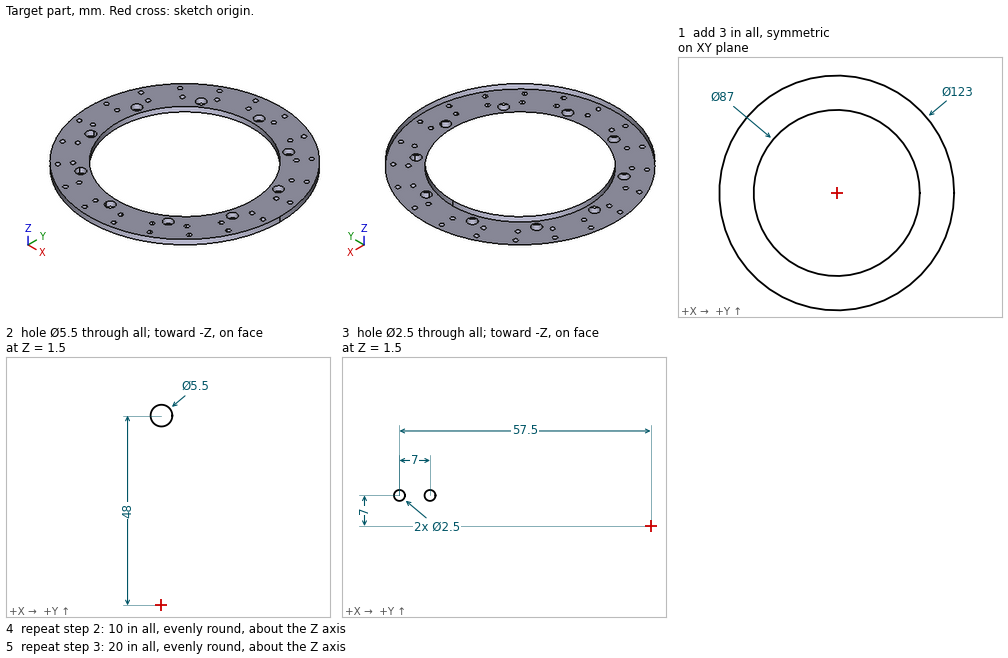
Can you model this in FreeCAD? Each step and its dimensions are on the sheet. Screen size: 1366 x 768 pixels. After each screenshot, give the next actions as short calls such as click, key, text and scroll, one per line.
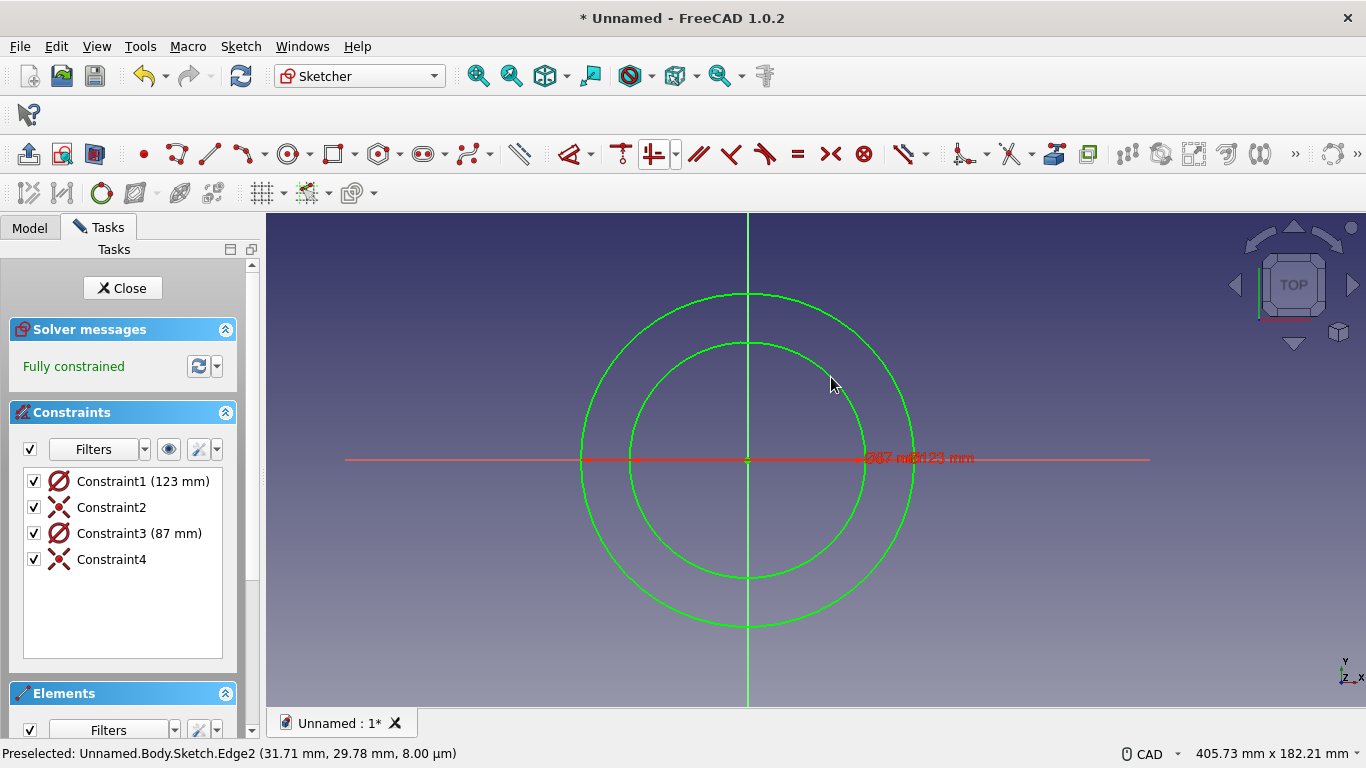
click(123, 288)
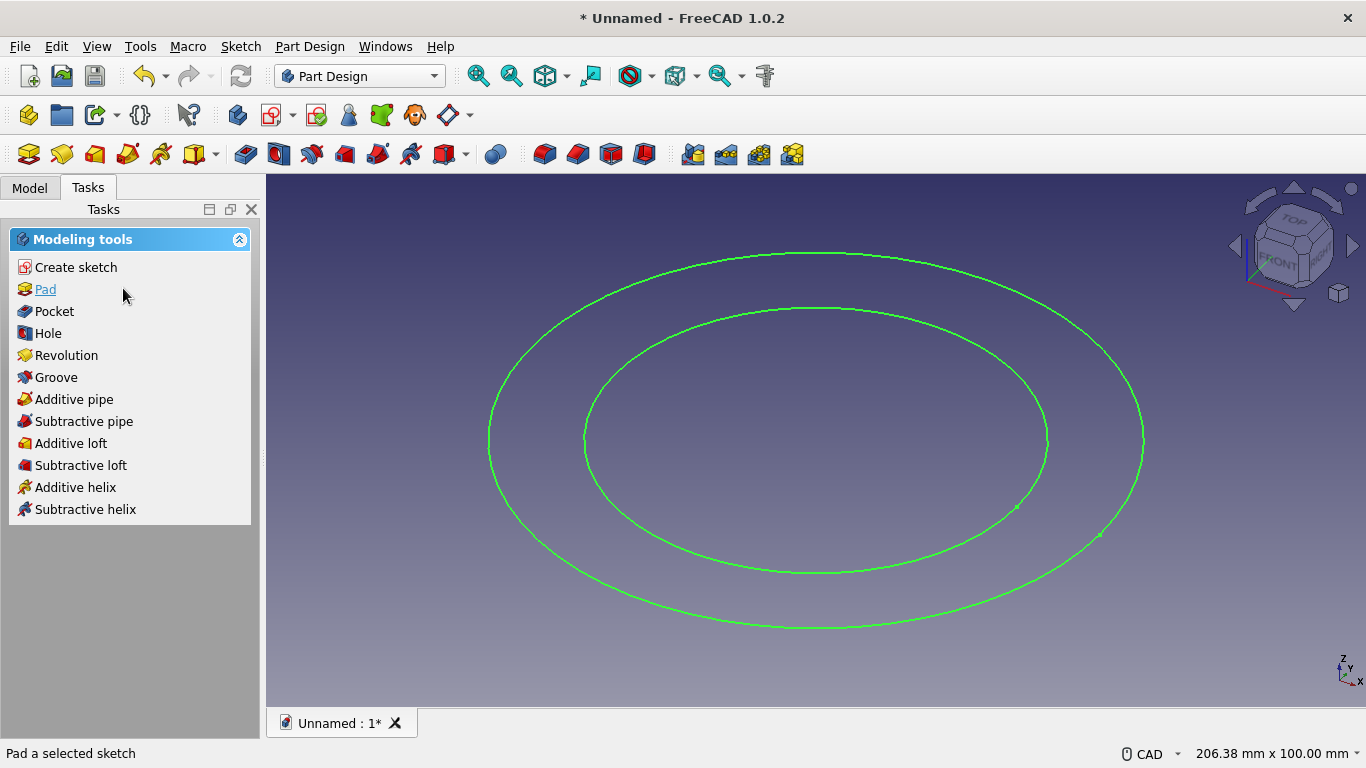
click(29, 154)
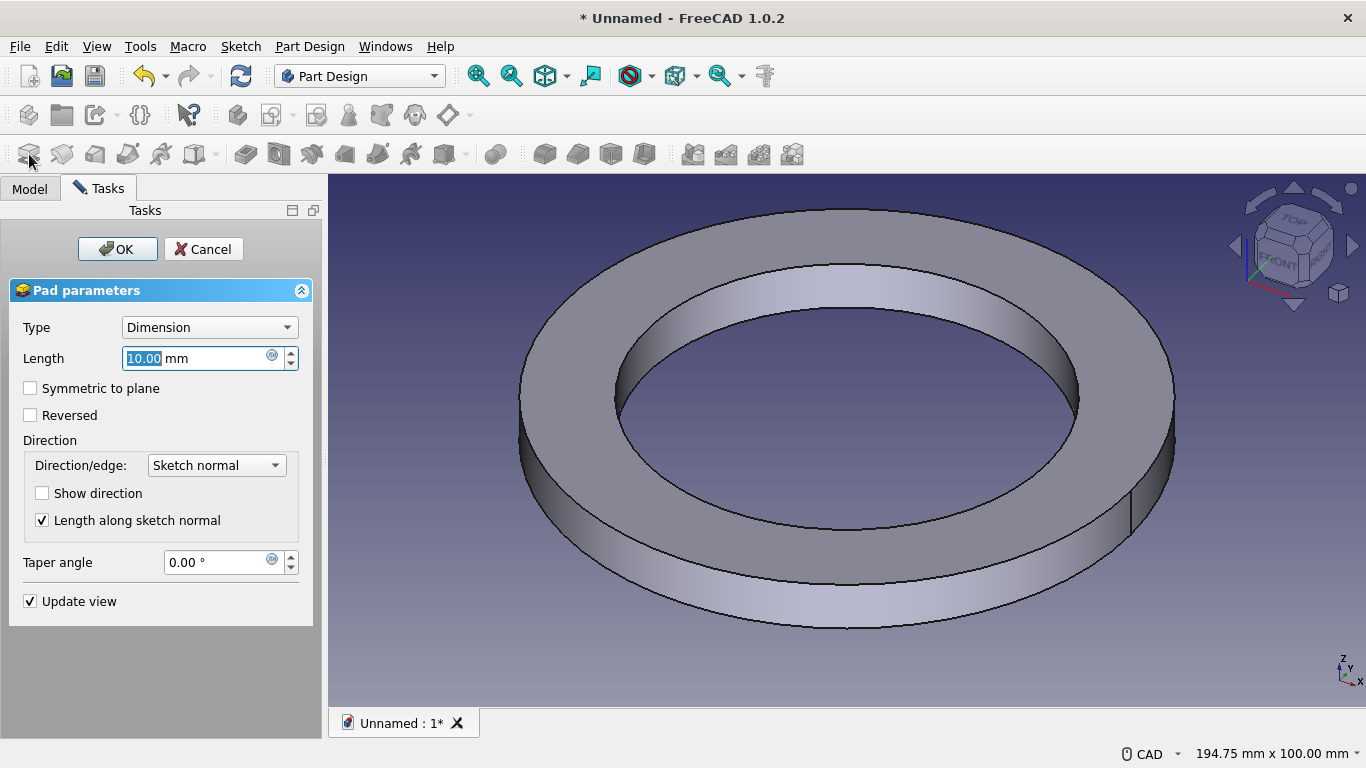
text(3)
key(Tab)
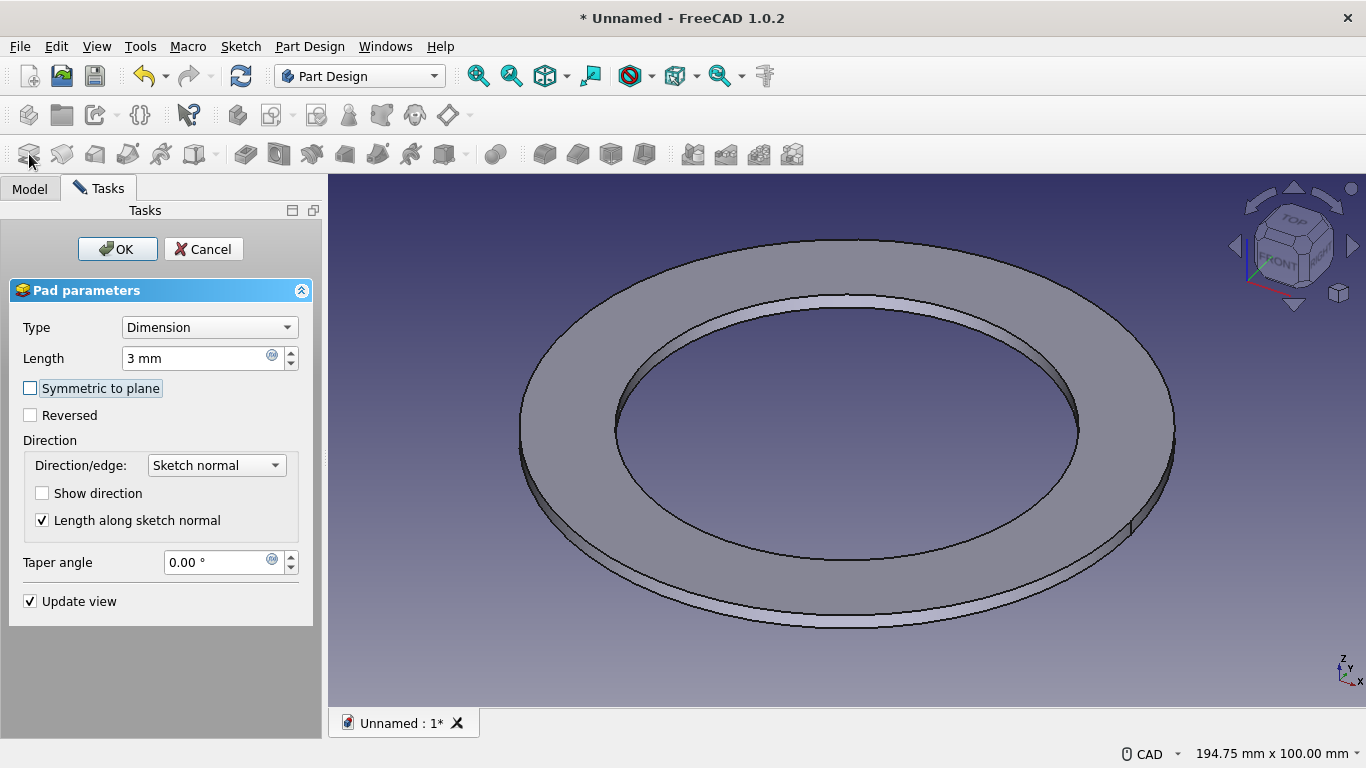
click(31, 388)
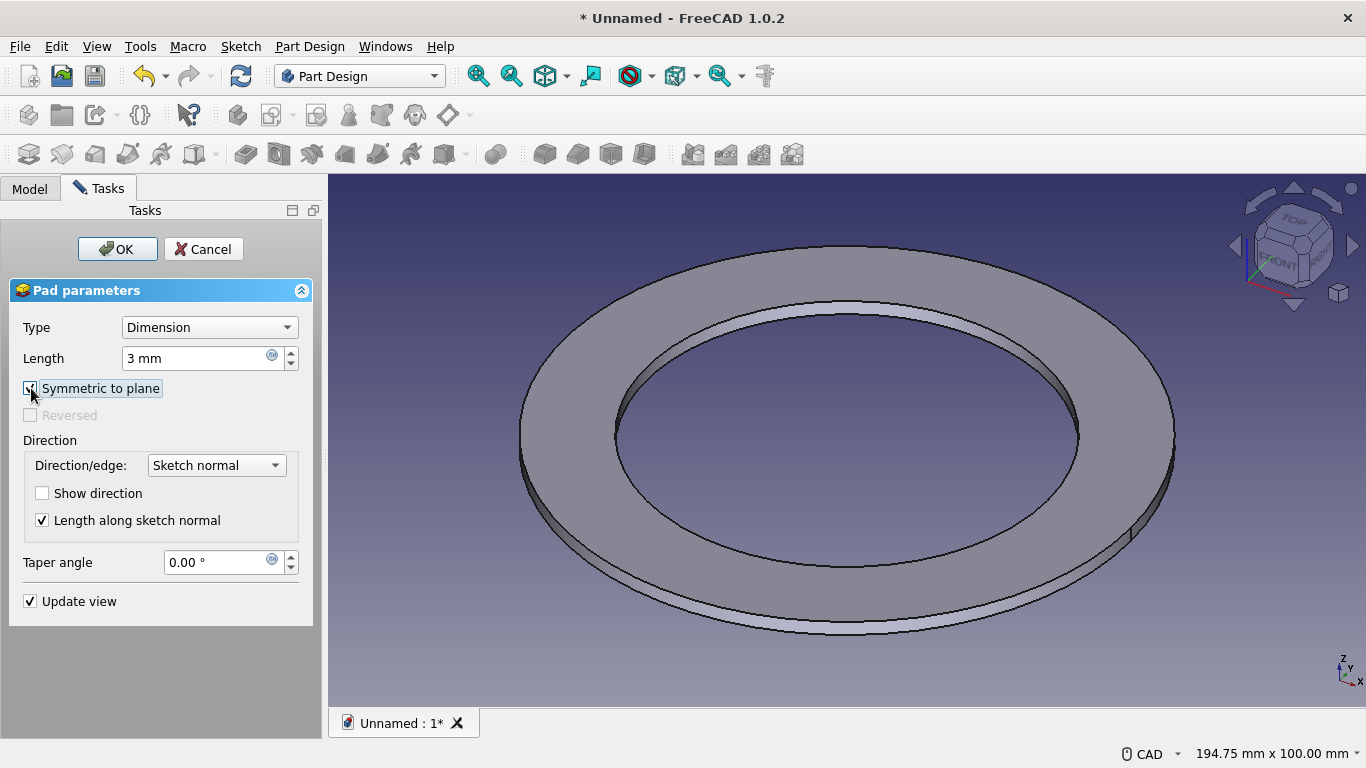
click(118, 249)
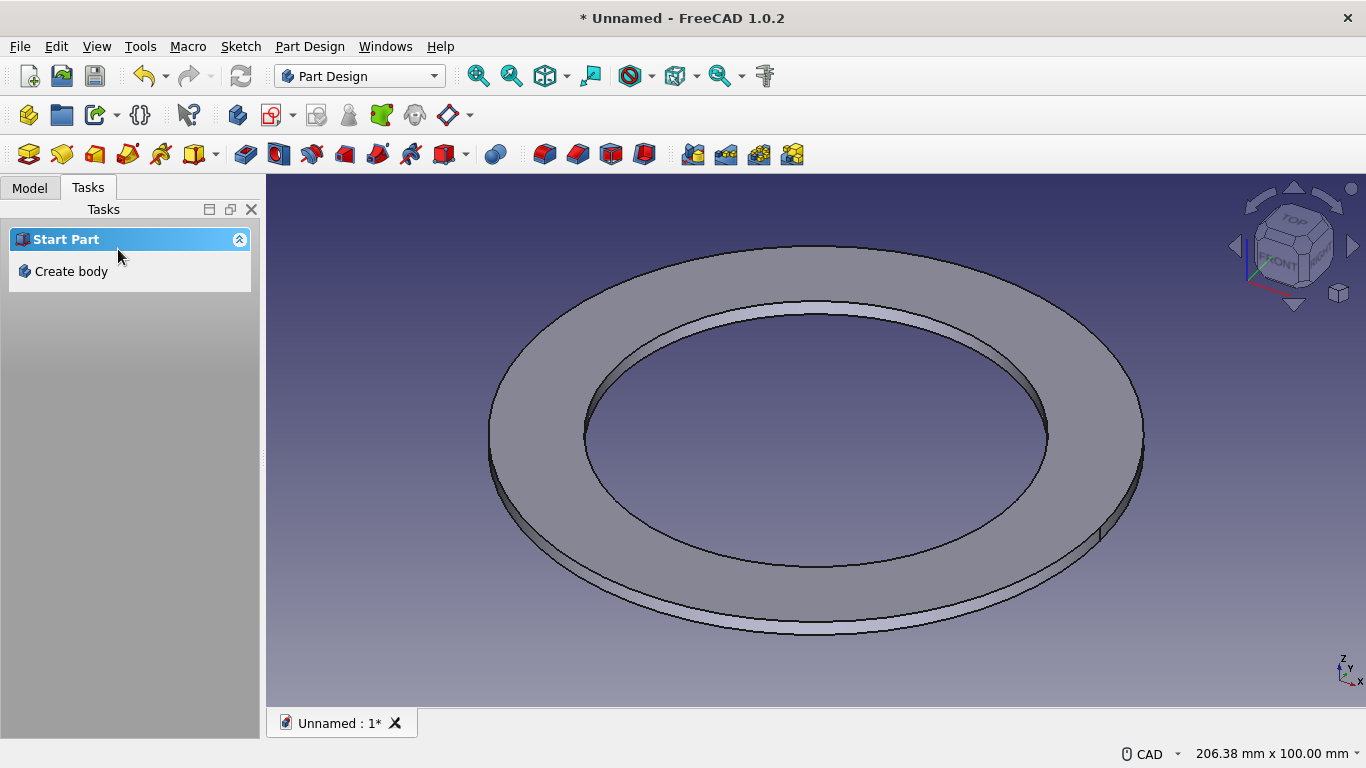
click(1059, 514)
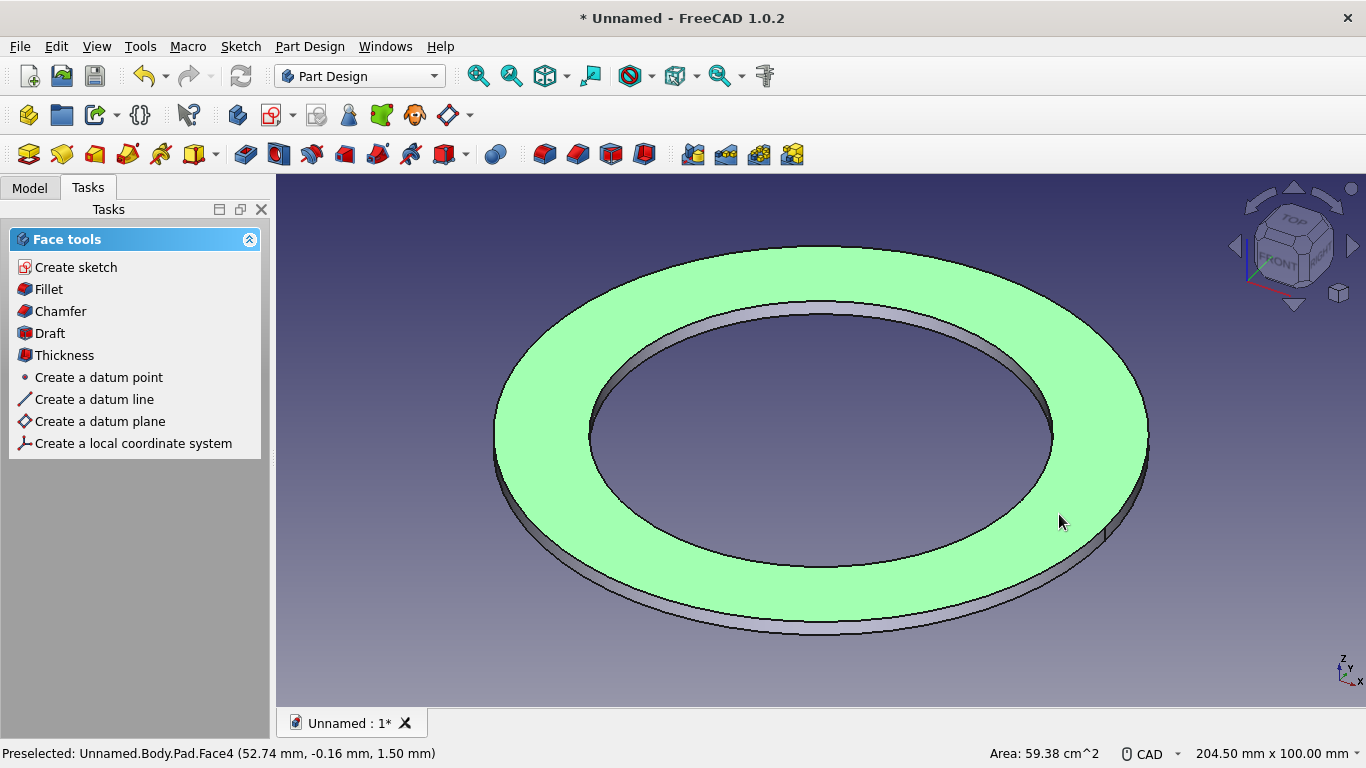
click(270, 116)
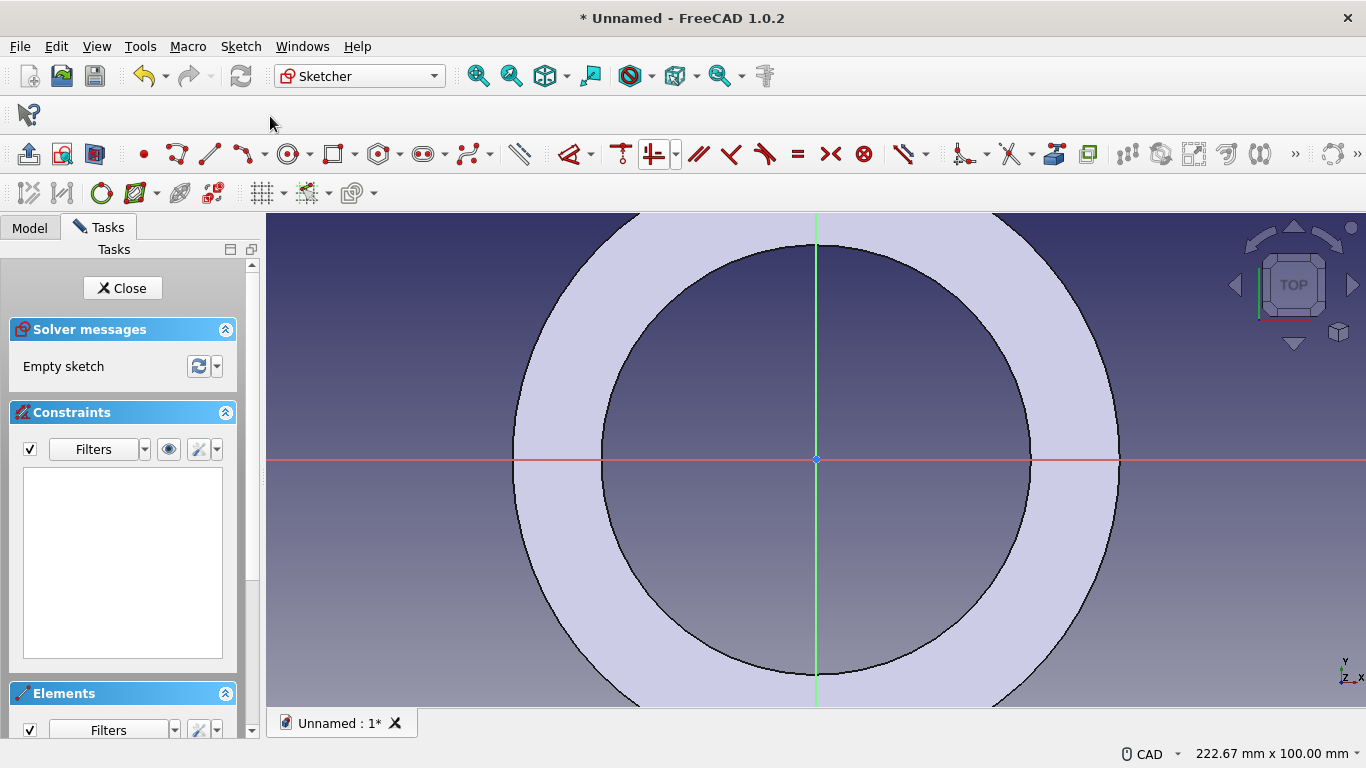
scroll(748, 460, down, 5)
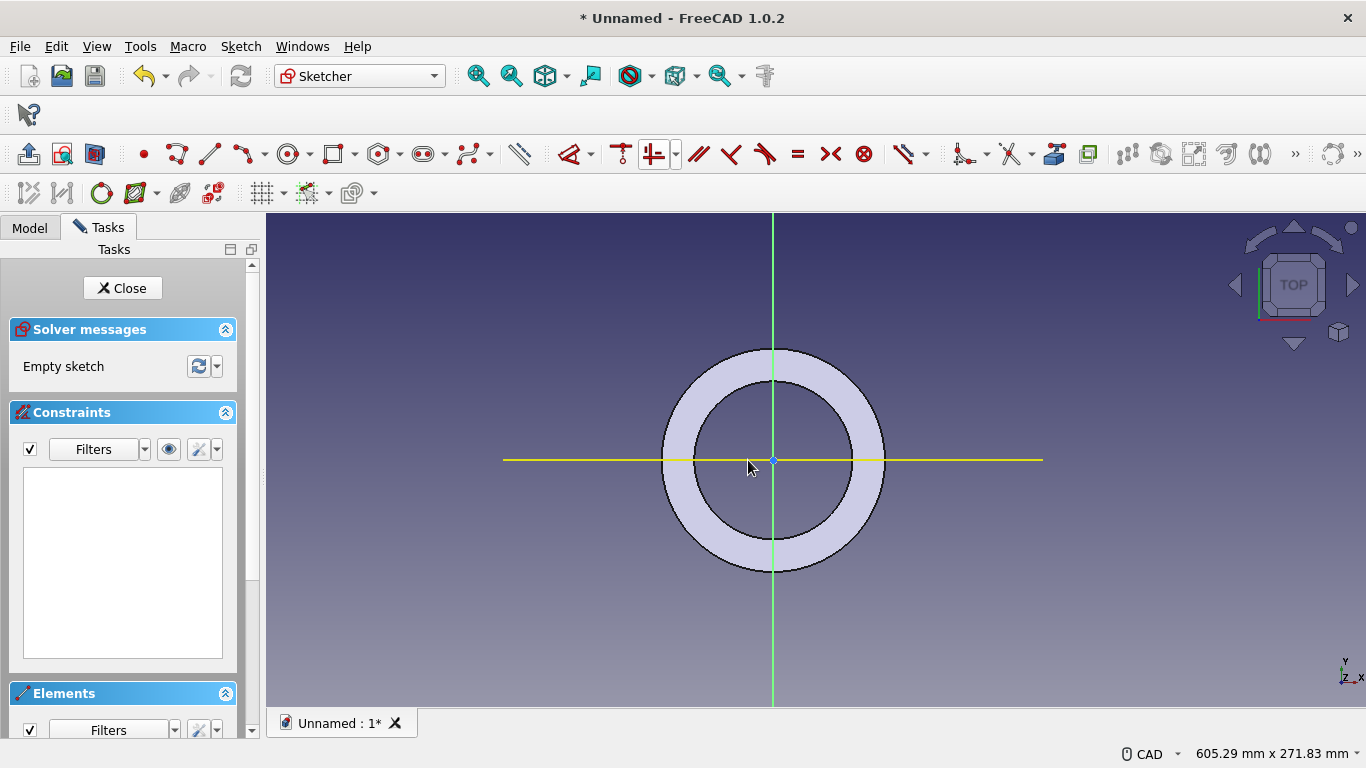
scroll(775, 369, up, 15)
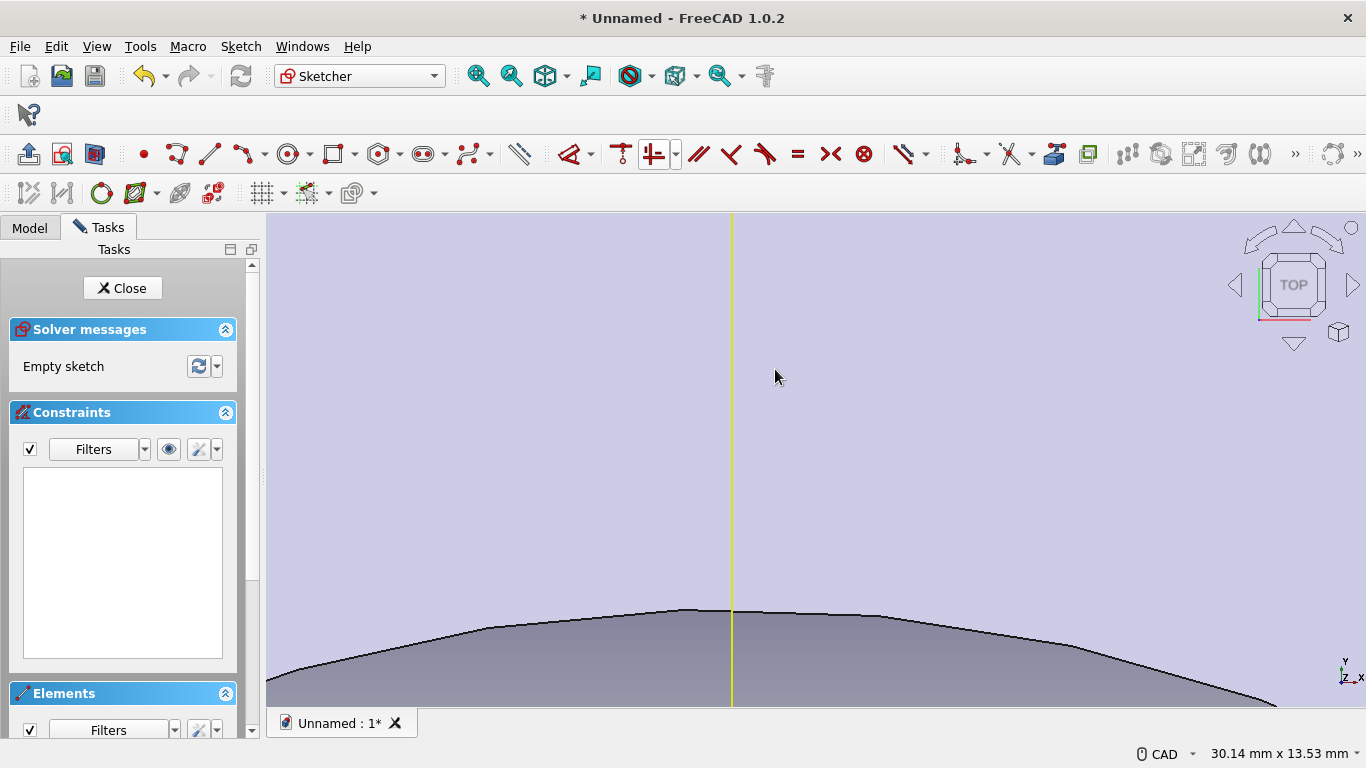
scroll(700, 415, up, 2)